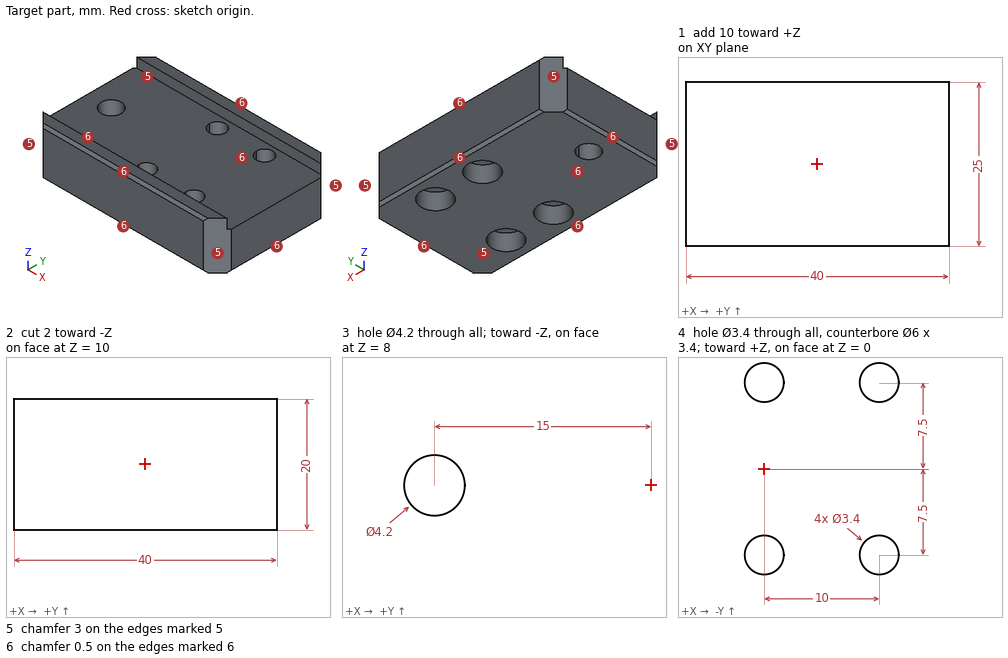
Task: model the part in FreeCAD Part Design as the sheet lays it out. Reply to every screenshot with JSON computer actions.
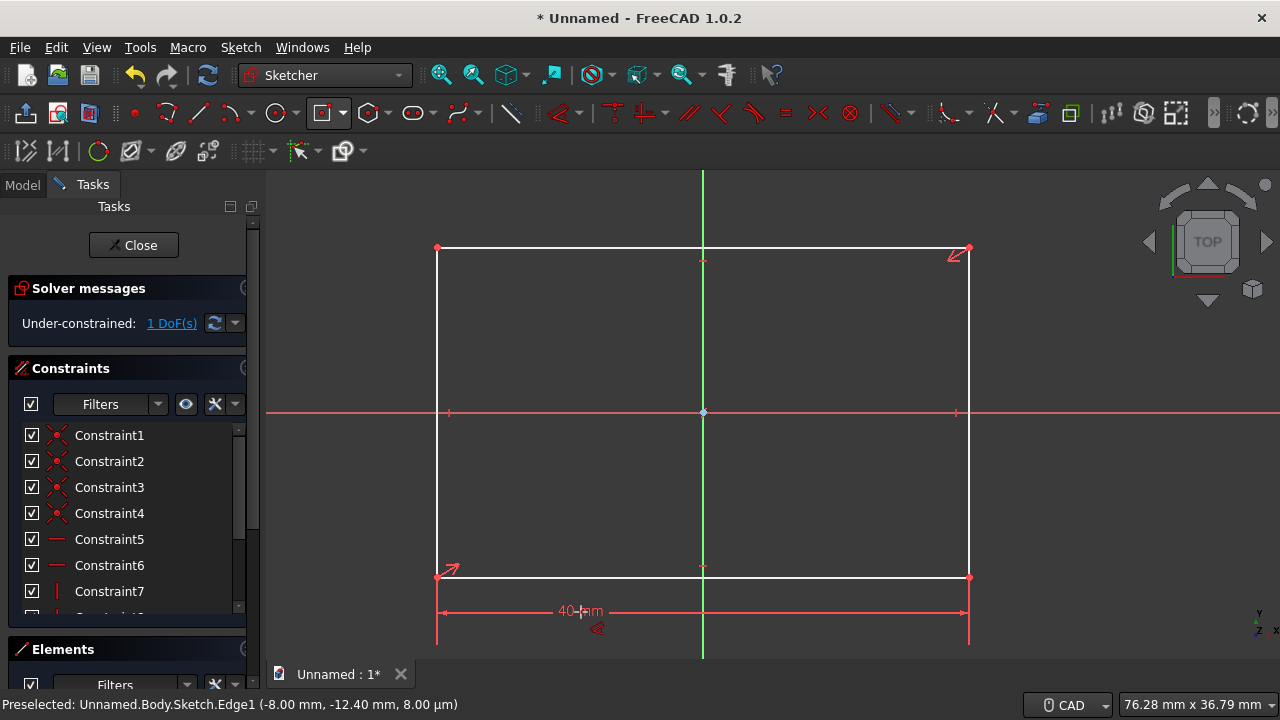
{"action": "left_click", "coordinate": [969, 479]}
{"action": "left_click", "coordinate": [1003, 337]}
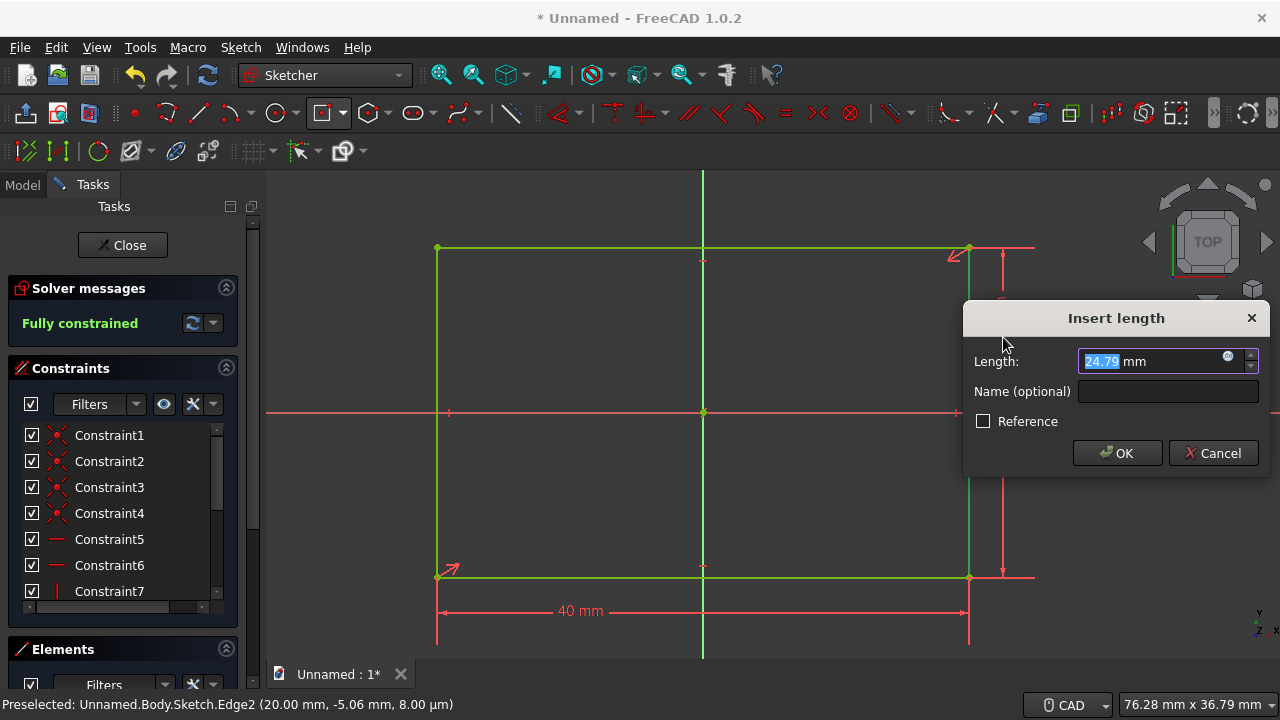
{"action": "type", "text": "25"}
{"action": "key", "text": "Return"}
{"action": "key", "text": "Escape"}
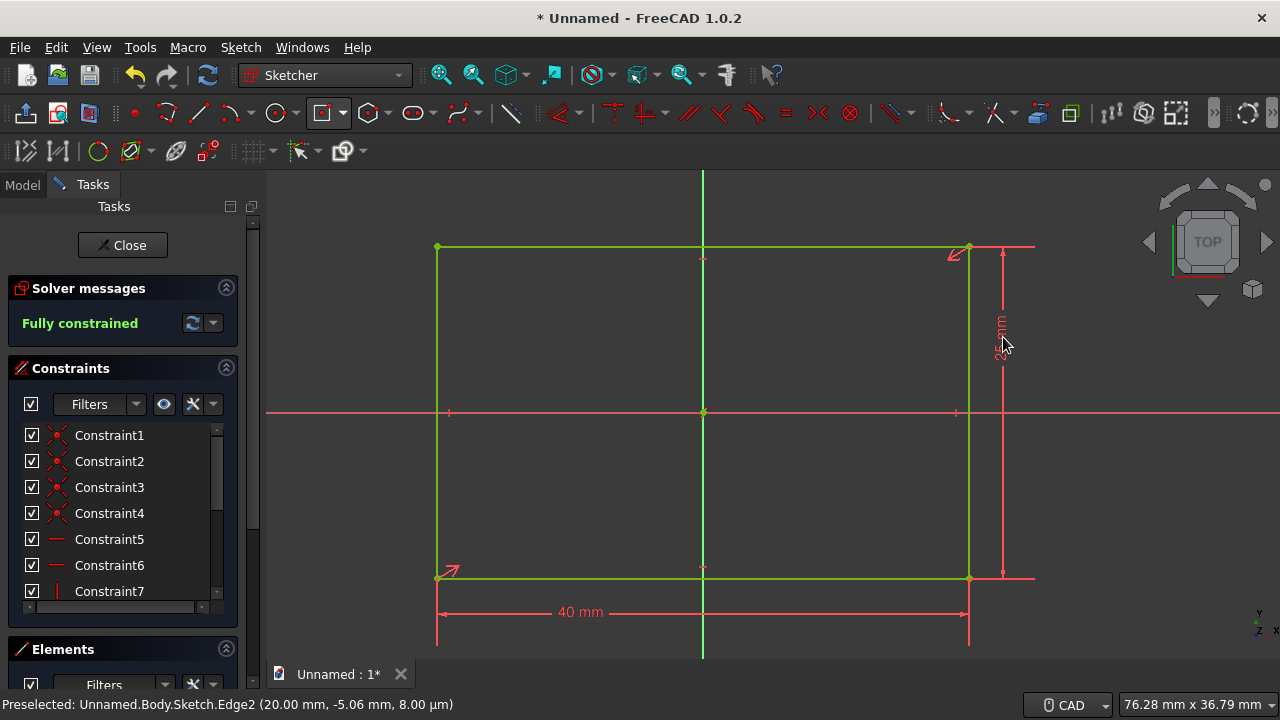
{"action": "left_click", "coordinate": [123, 245]}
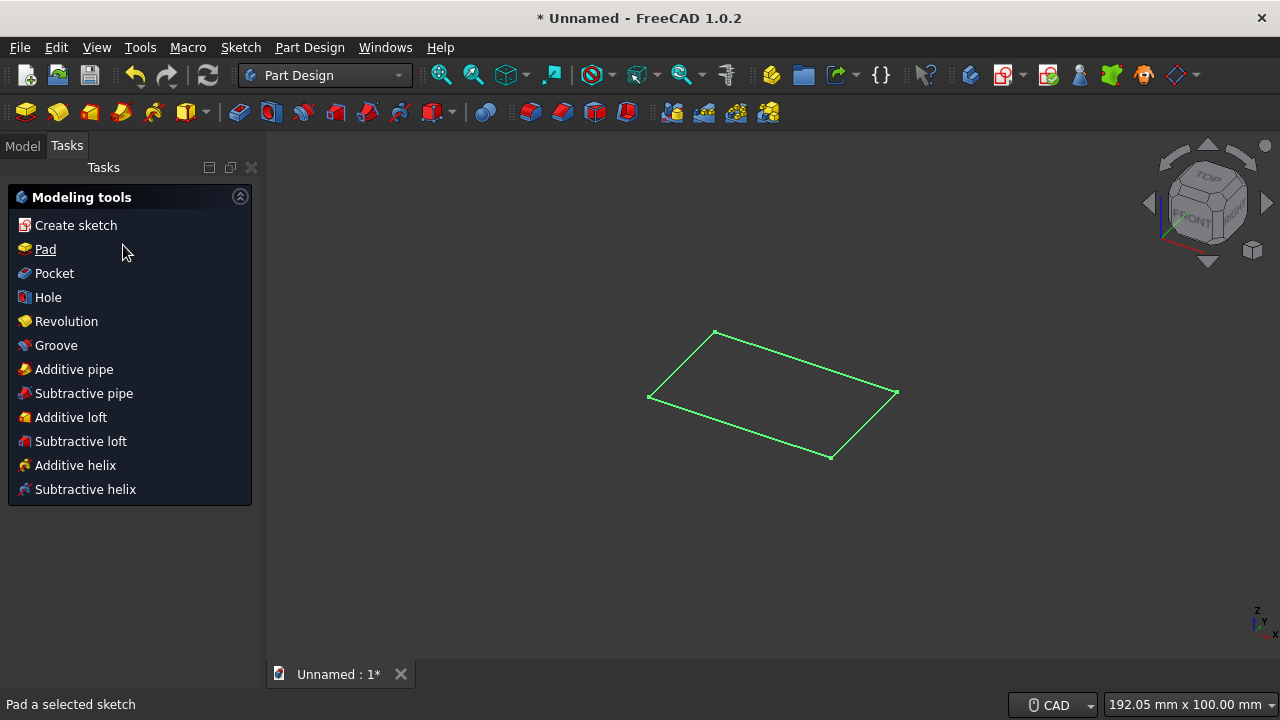
{"action": "left_click", "coordinate": [26, 112]}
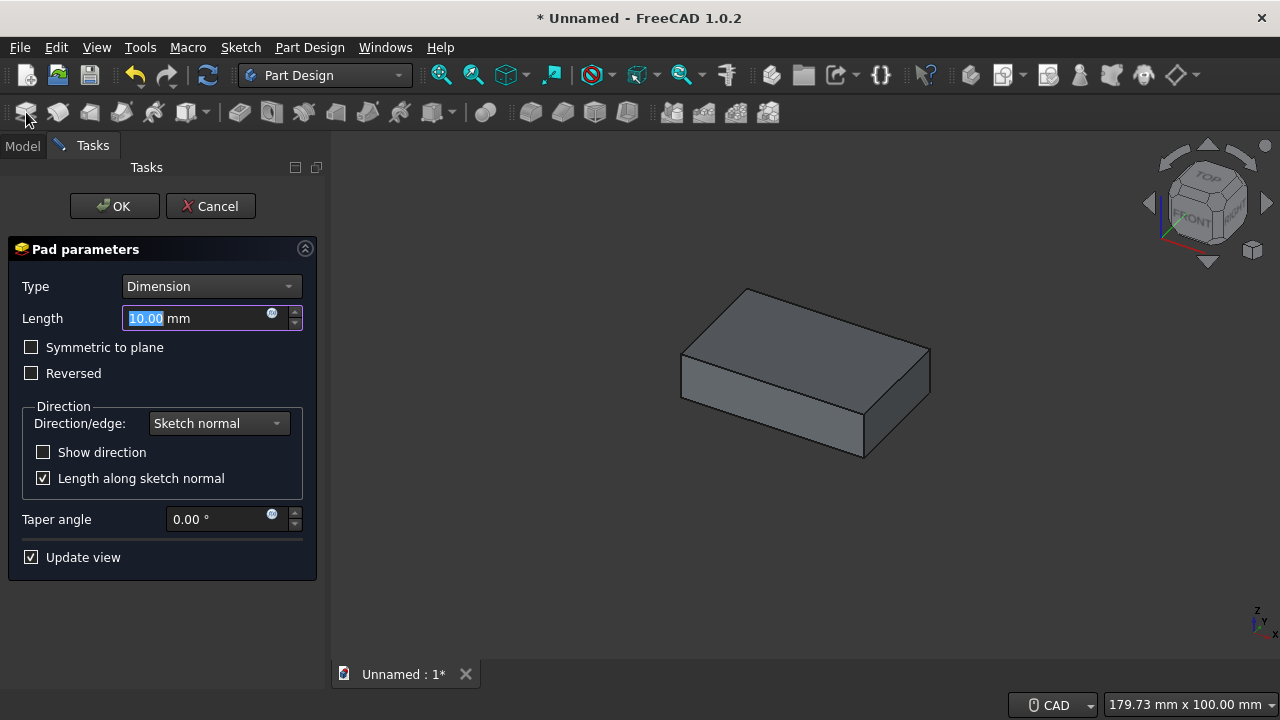
{"action": "type", "text": "10"}
{"action": "key", "text": "Tab"}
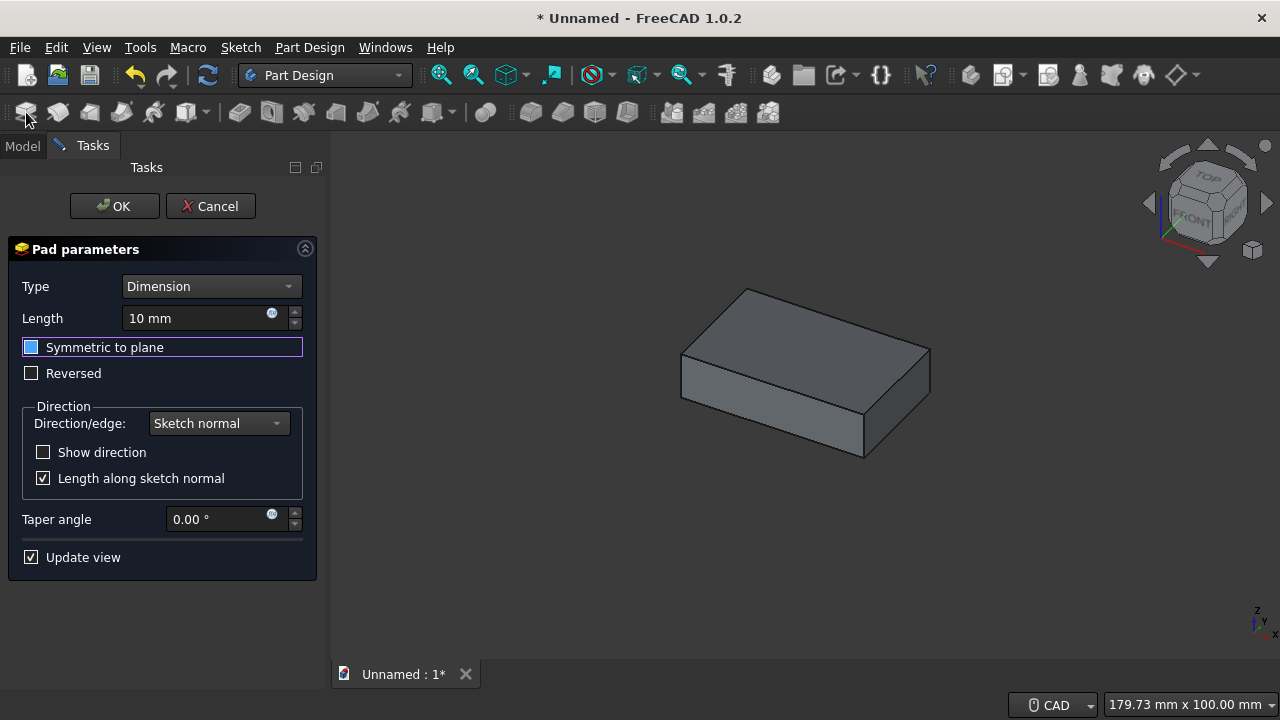
{"action": "left_click", "coordinate": [115, 206]}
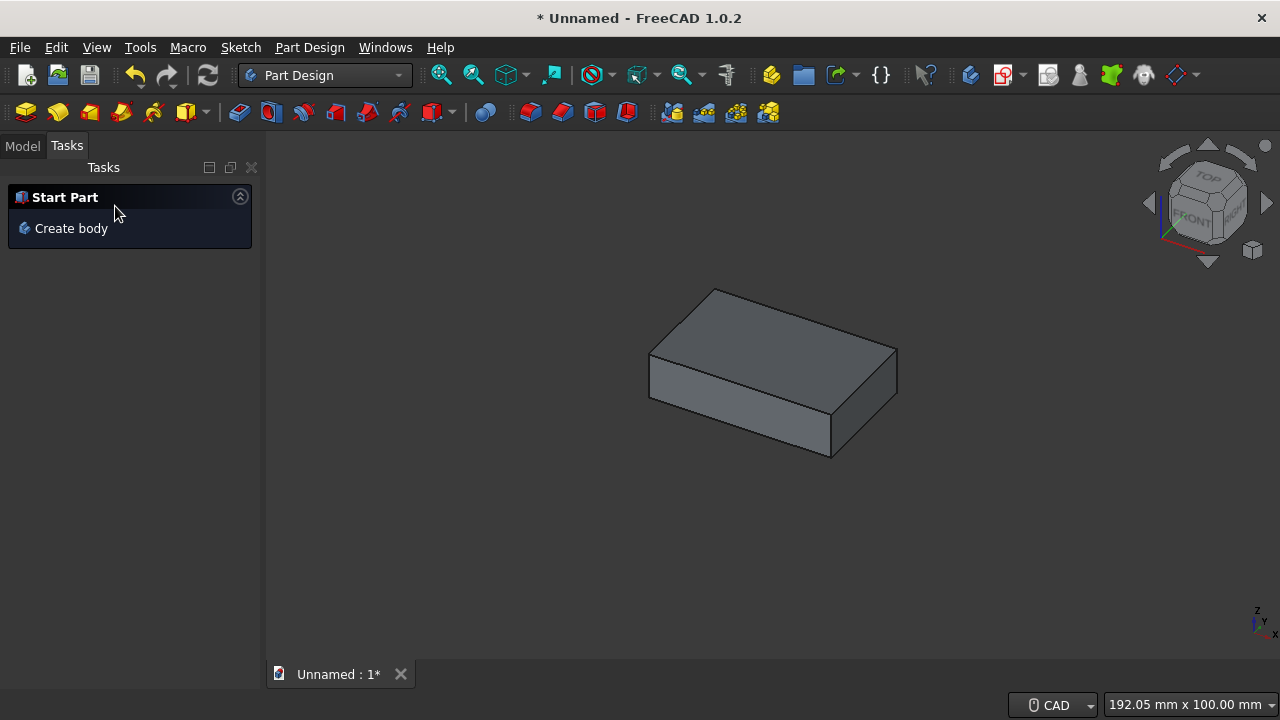
{"action": "left_click", "coordinate": [442, 76]}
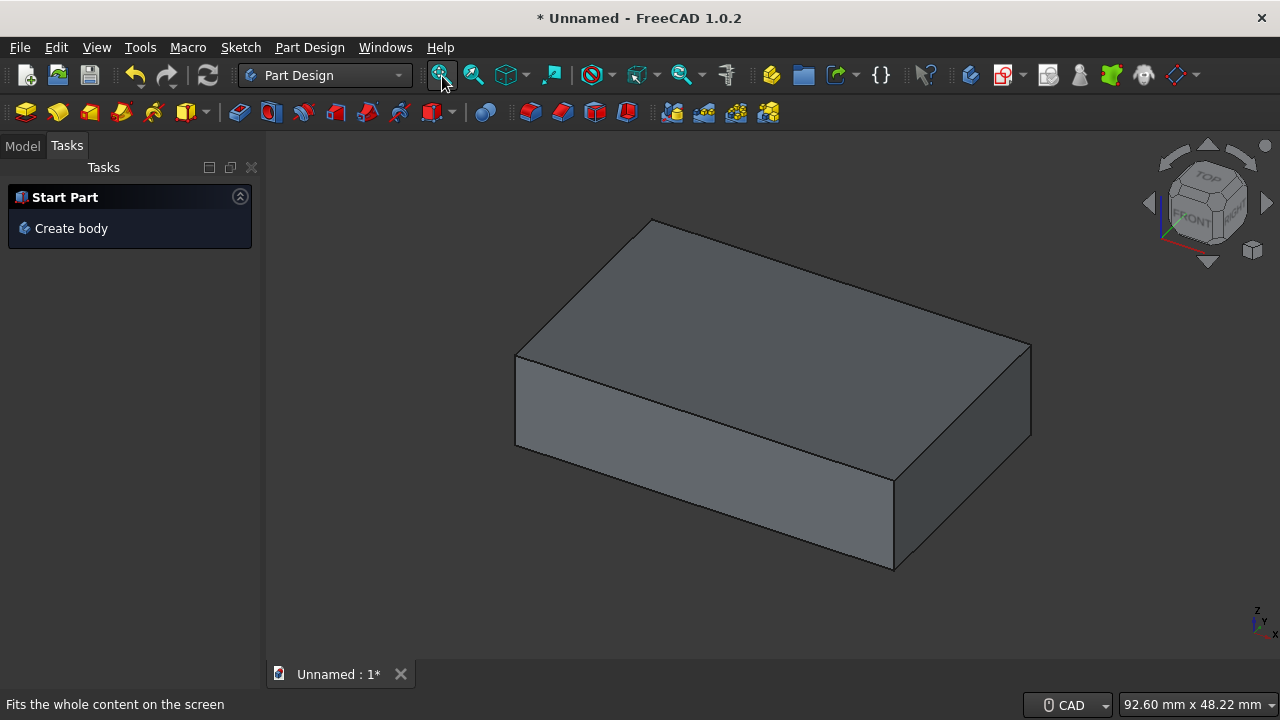
{"action": "left_click", "coordinate": [827, 367]}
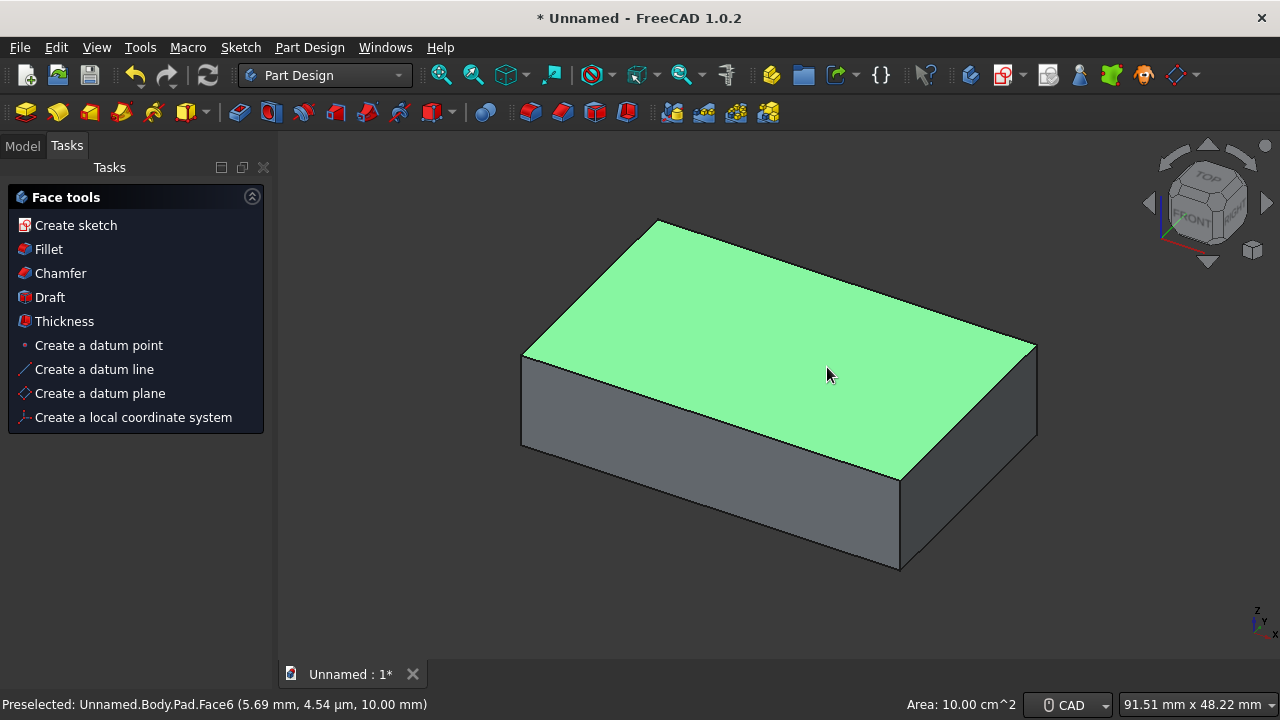
{"action": "left_click", "coordinate": [1004, 76]}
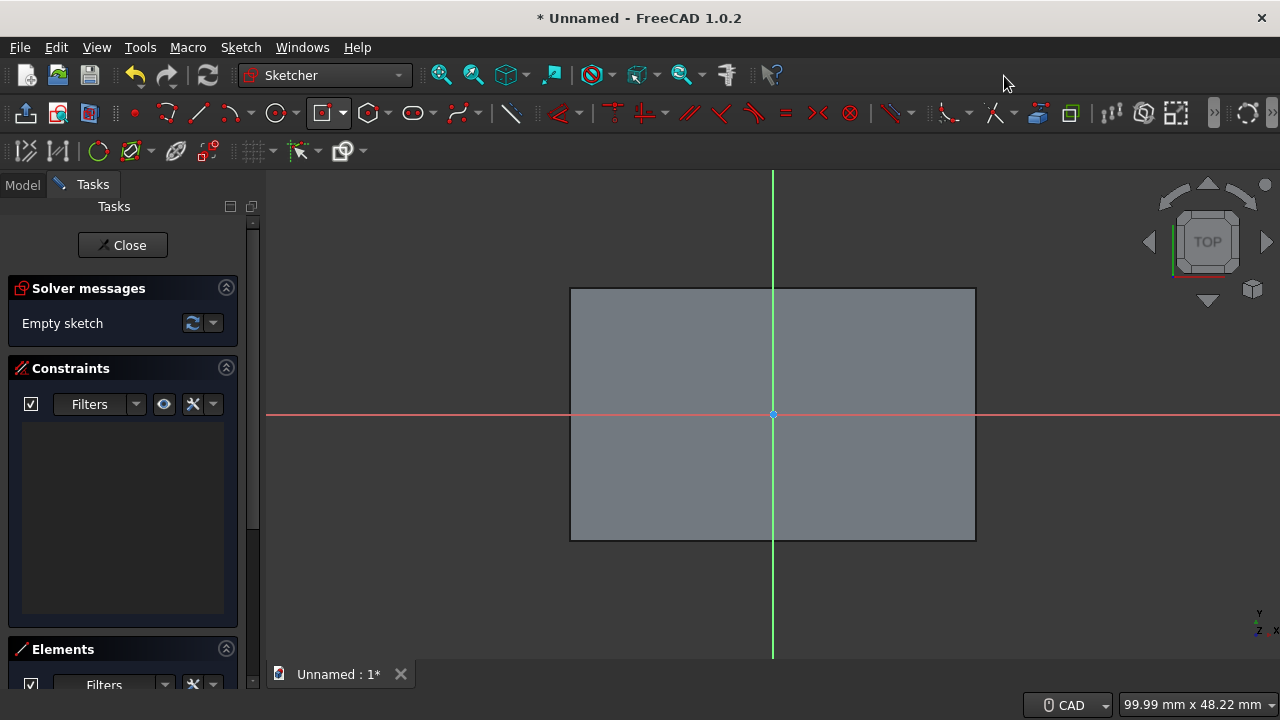
{"action": "scroll", "coordinate": [912, 414], "scroll_direction": "up", "scroll_amount": 2}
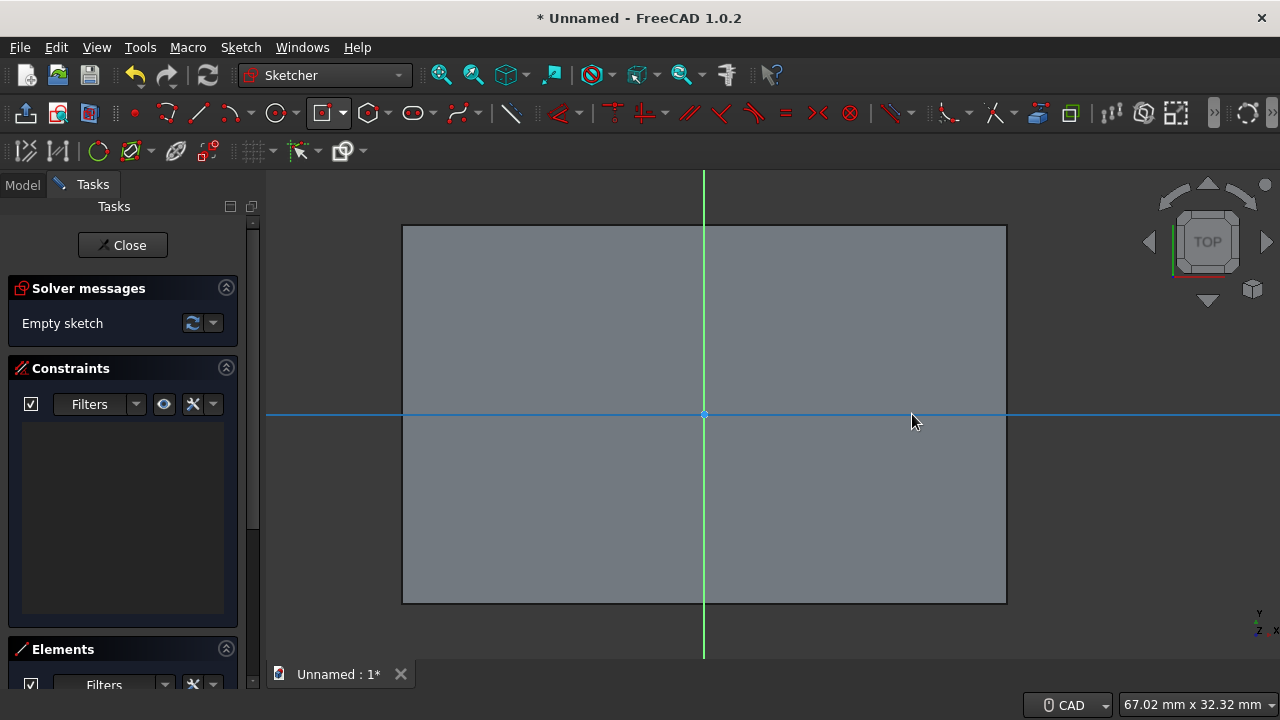
{"action": "left_click", "coordinate": [322, 114]}